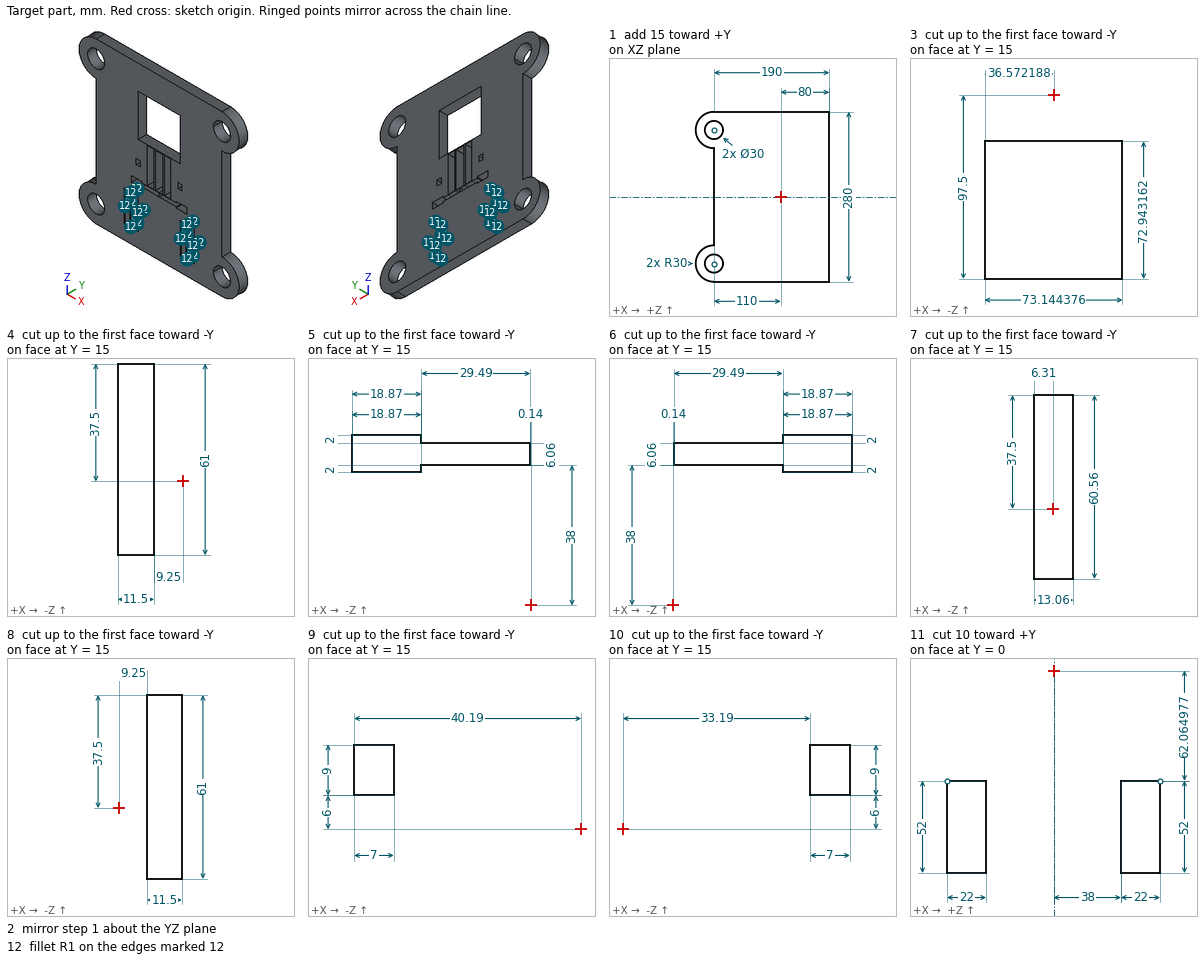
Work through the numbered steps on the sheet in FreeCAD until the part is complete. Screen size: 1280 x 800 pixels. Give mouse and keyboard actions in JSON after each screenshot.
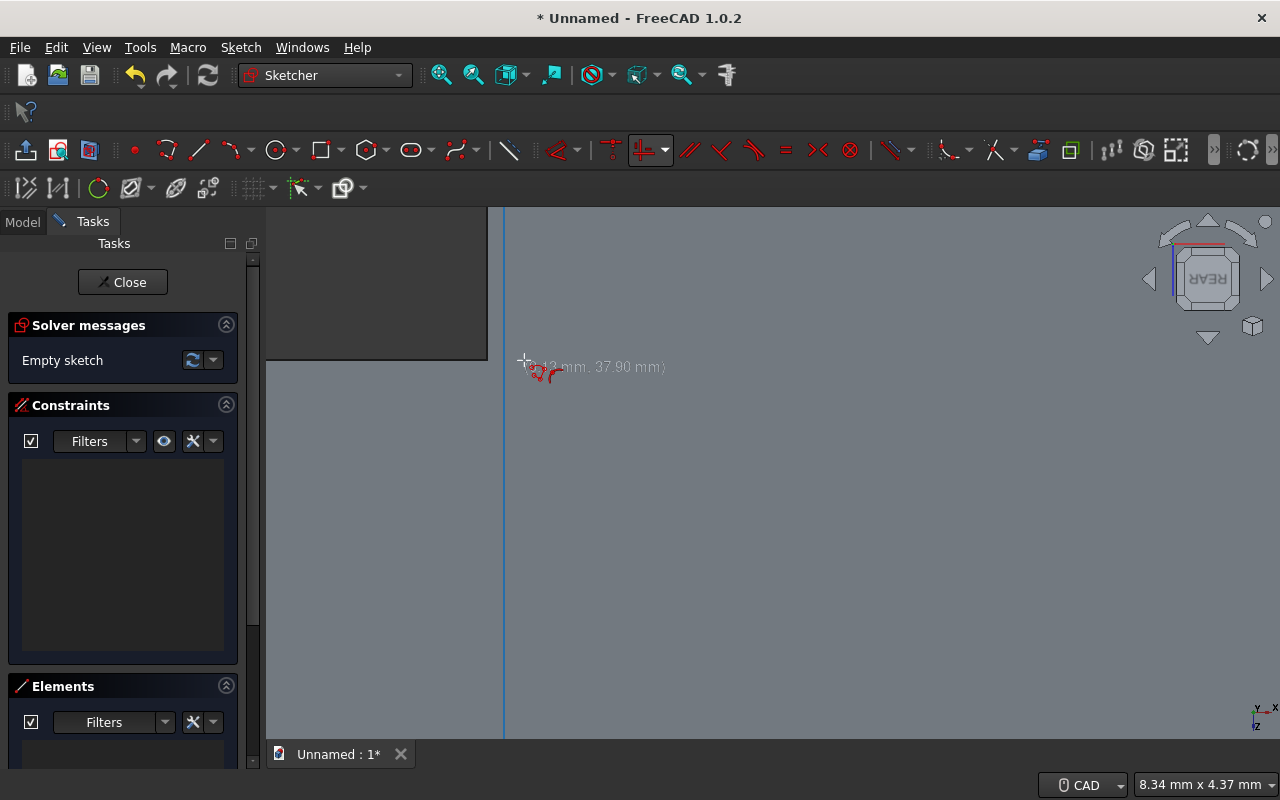
{"action": "left_click", "coordinate": [521, 360]}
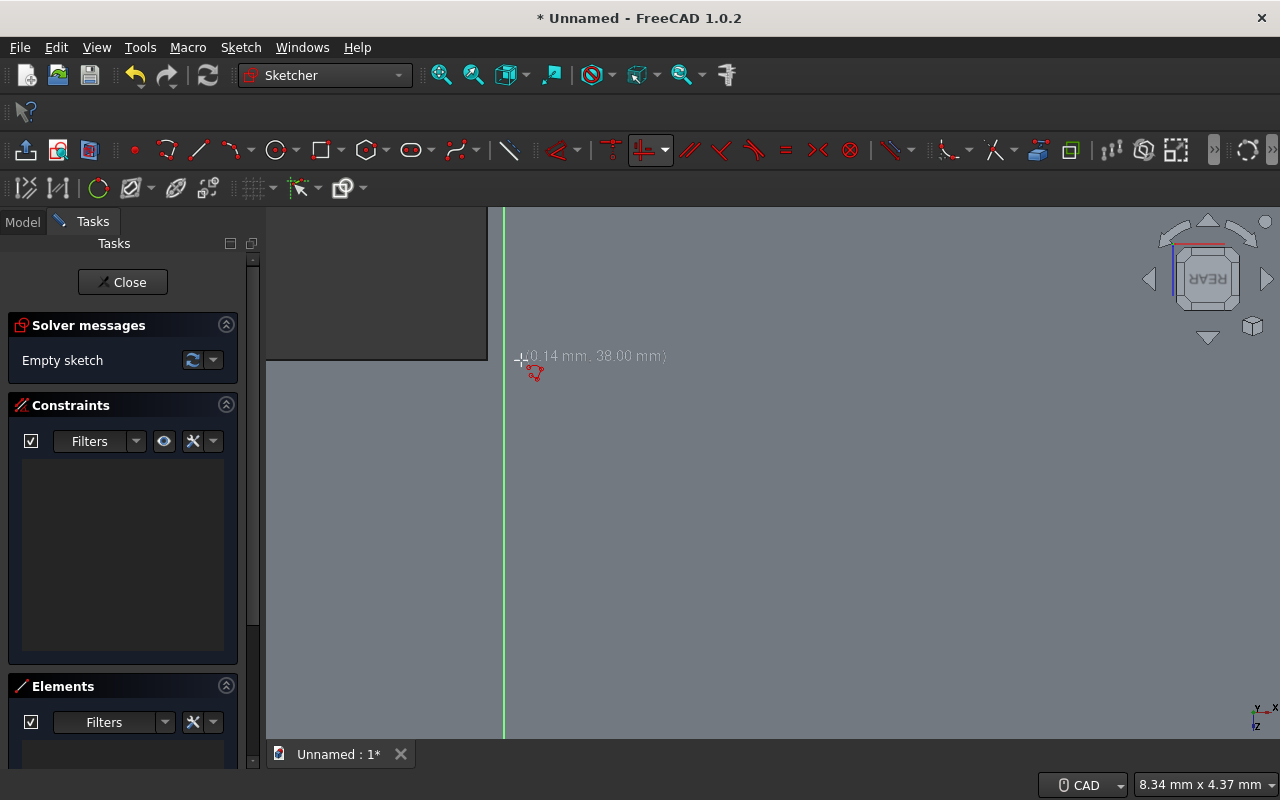
{"action": "scroll", "coordinate": [527, 362], "scroll_direction": "down", "scroll_amount": 14}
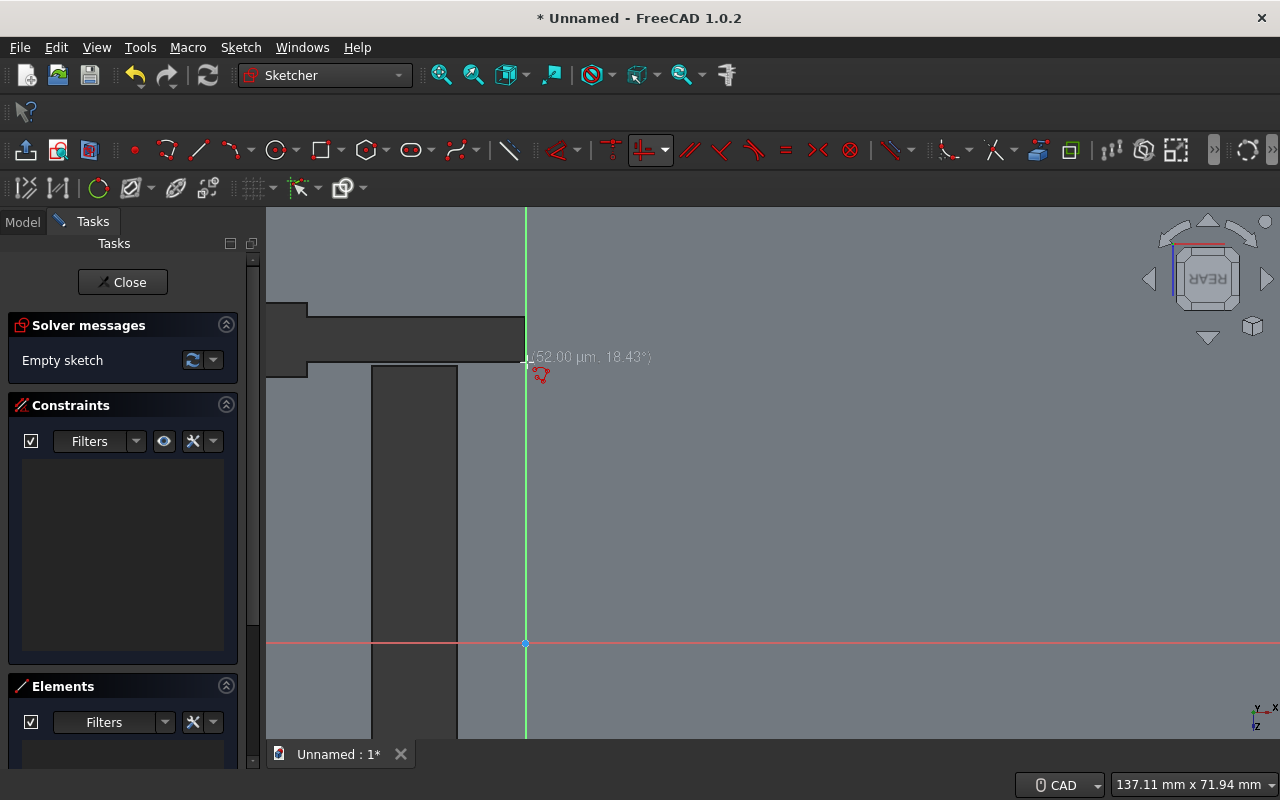
{"action": "left_click", "coordinate": [745, 362]}
{"action": "left_click", "coordinate": [745, 377]}
{"action": "left_click", "coordinate": [885, 377]}
{"action": "left_click", "coordinate": [885, 303]}
{"action": "left_click", "coordinate": [745, 303]}
{"action": "left_click", "coordinate": [745, 317]}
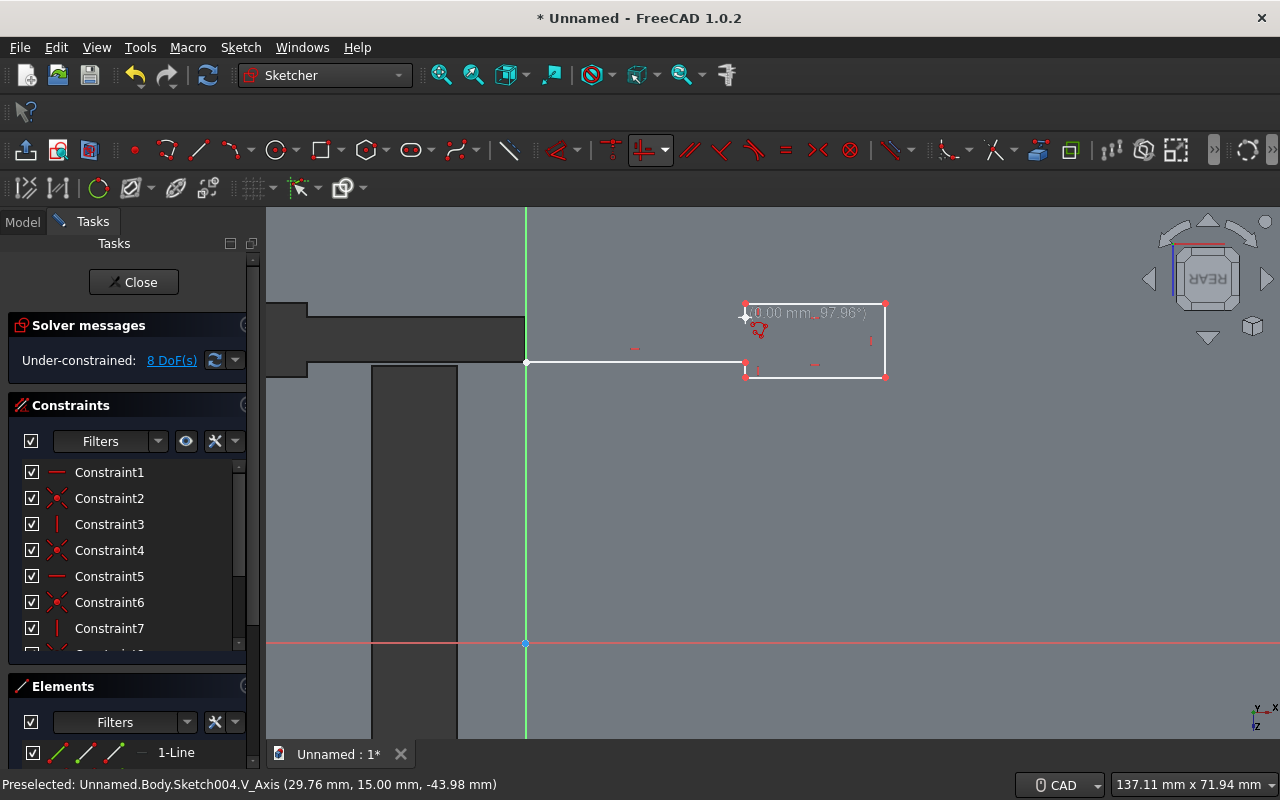
{"action": "scroll", "coordinate": [527, 317], "scroll_direction": "up", "scroll_amount": 14}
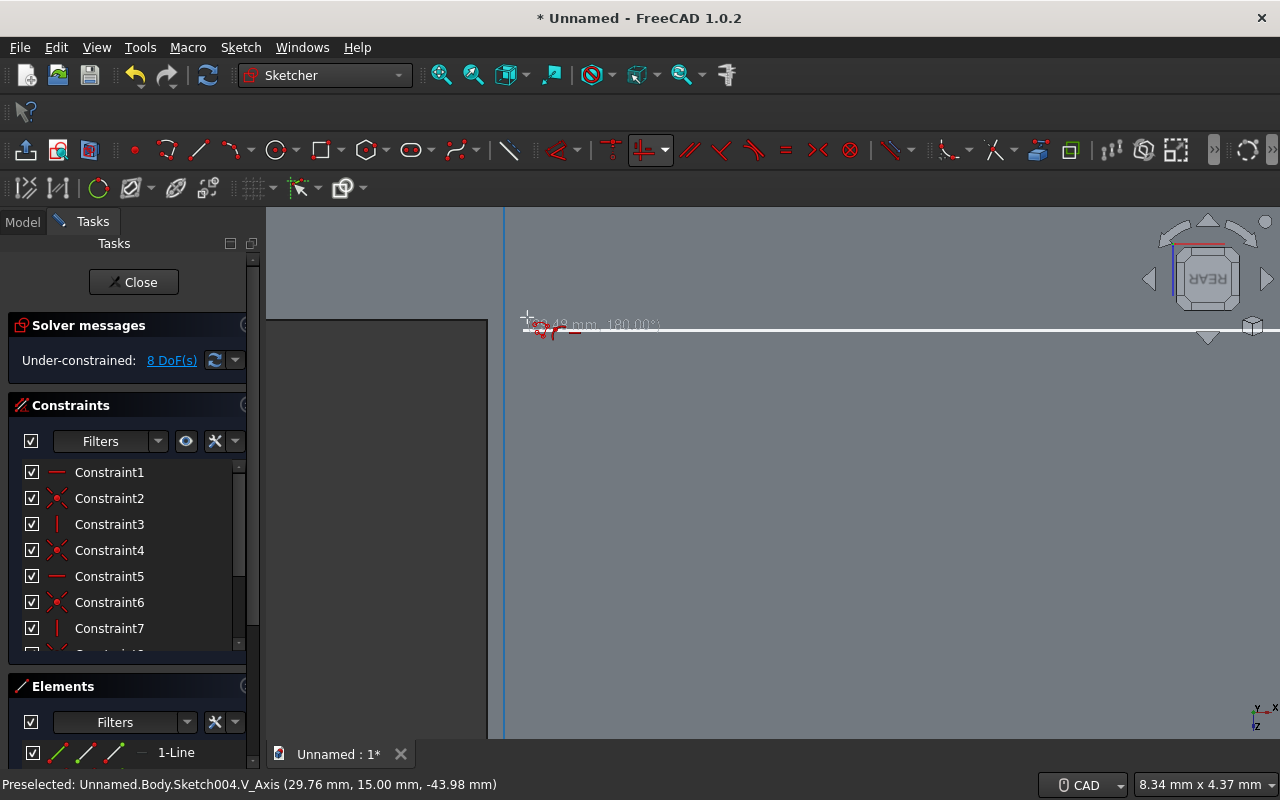
{"action": "left_click", "coordinate": [521, 314]}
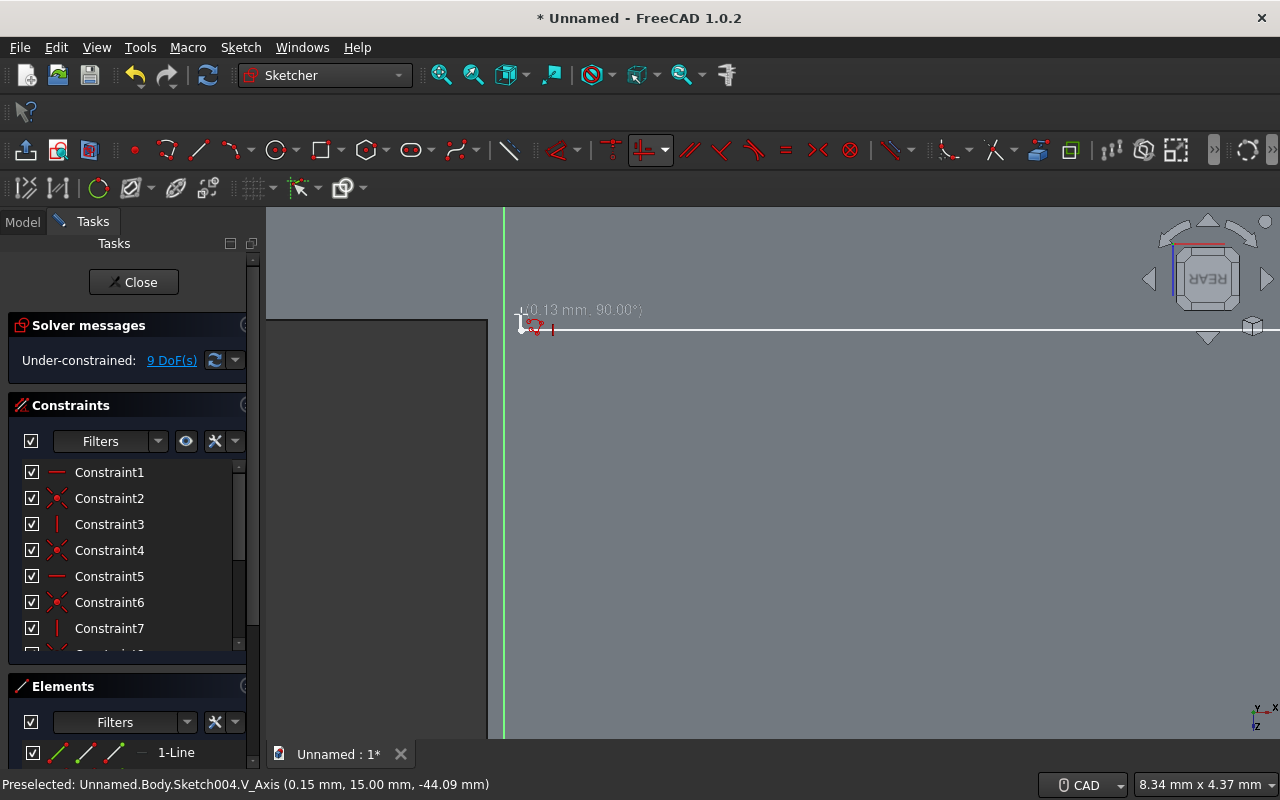
{"action": "scroll", "coordinate": [527, 317], "scroll_direction": "down", "scroll_amount": 14}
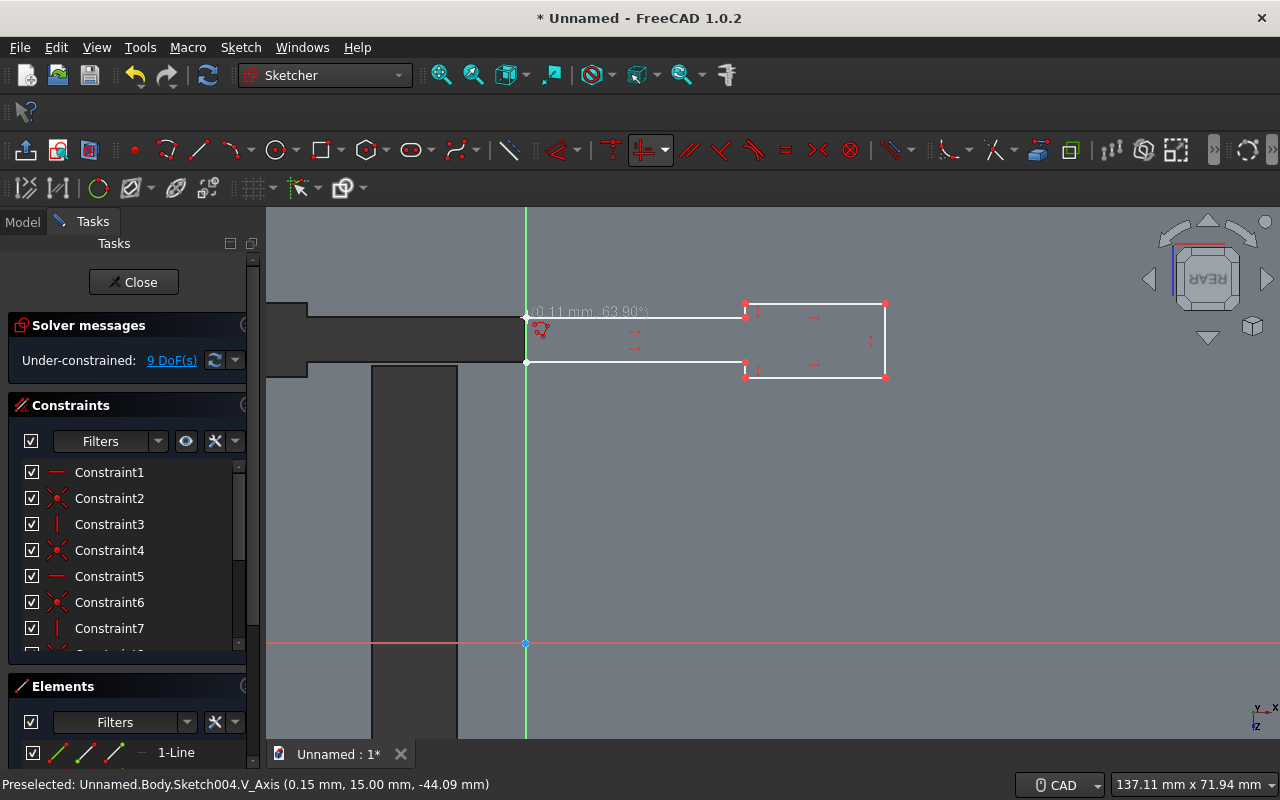
{"action": "scroll", "coordinate": [527, 362], "scroll_direction": "up", "scroll_amount": 14}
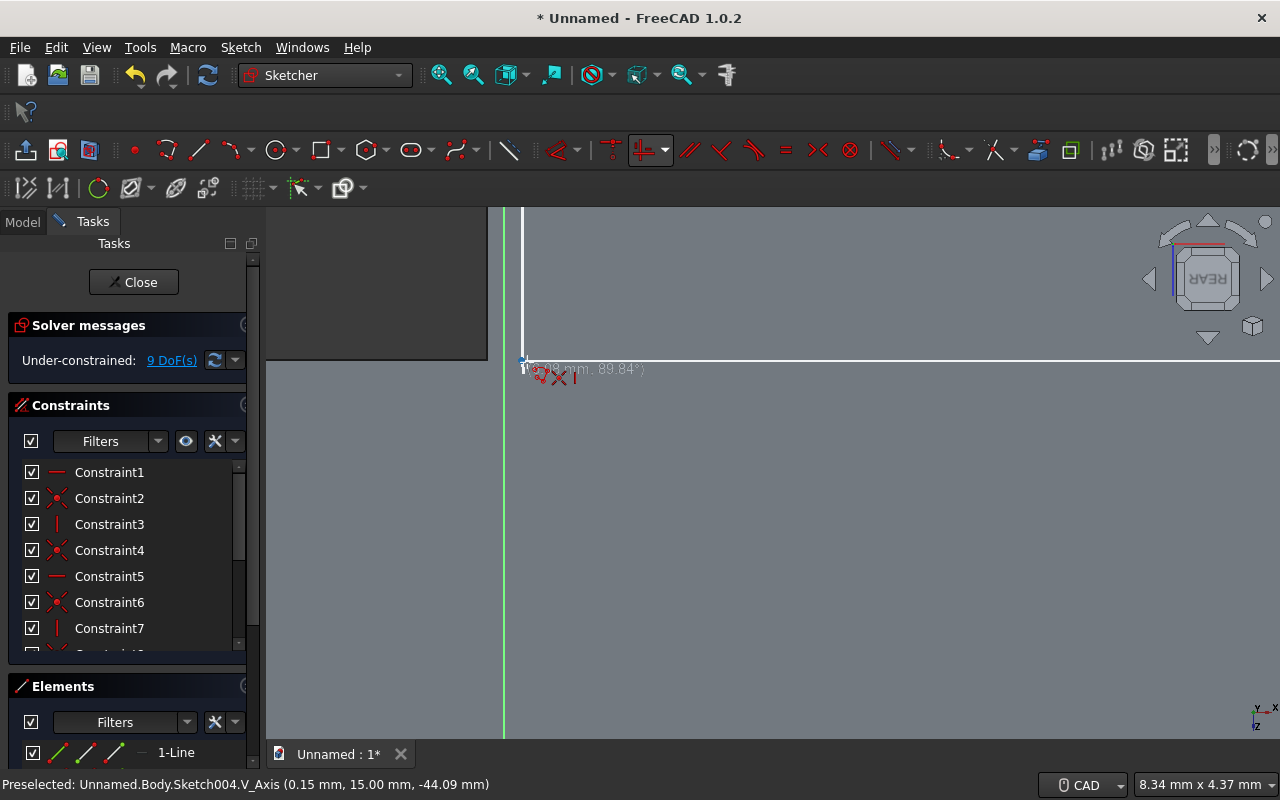
{"action": "left_click", "coordinate": [521, 361]}
{"action": "key", "text": "Escape"}
{"action": "key", "text": "Escape"}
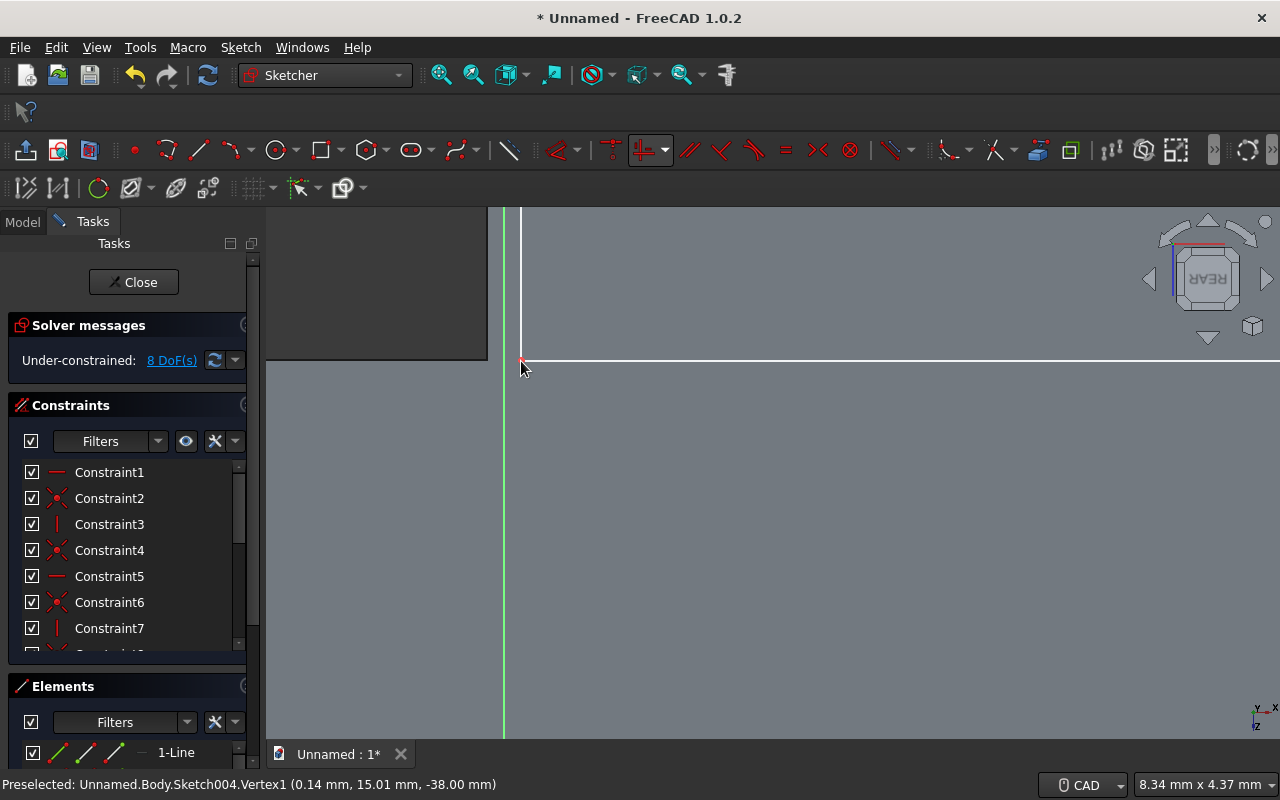
{"action": "left_click", "coordinate": [556, 150]}